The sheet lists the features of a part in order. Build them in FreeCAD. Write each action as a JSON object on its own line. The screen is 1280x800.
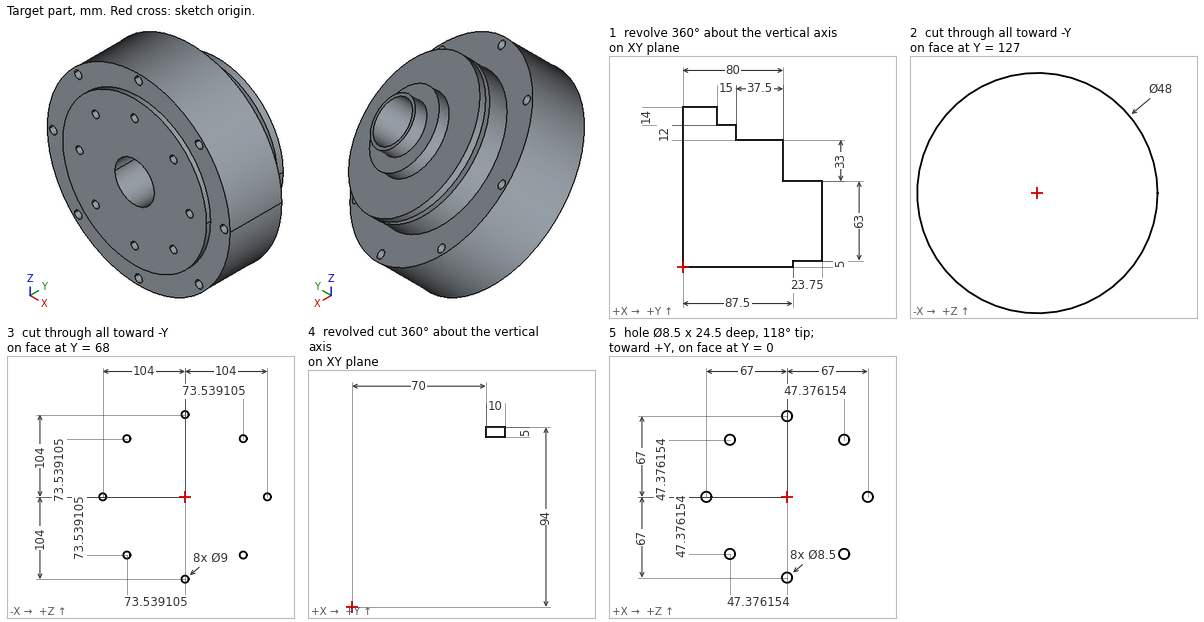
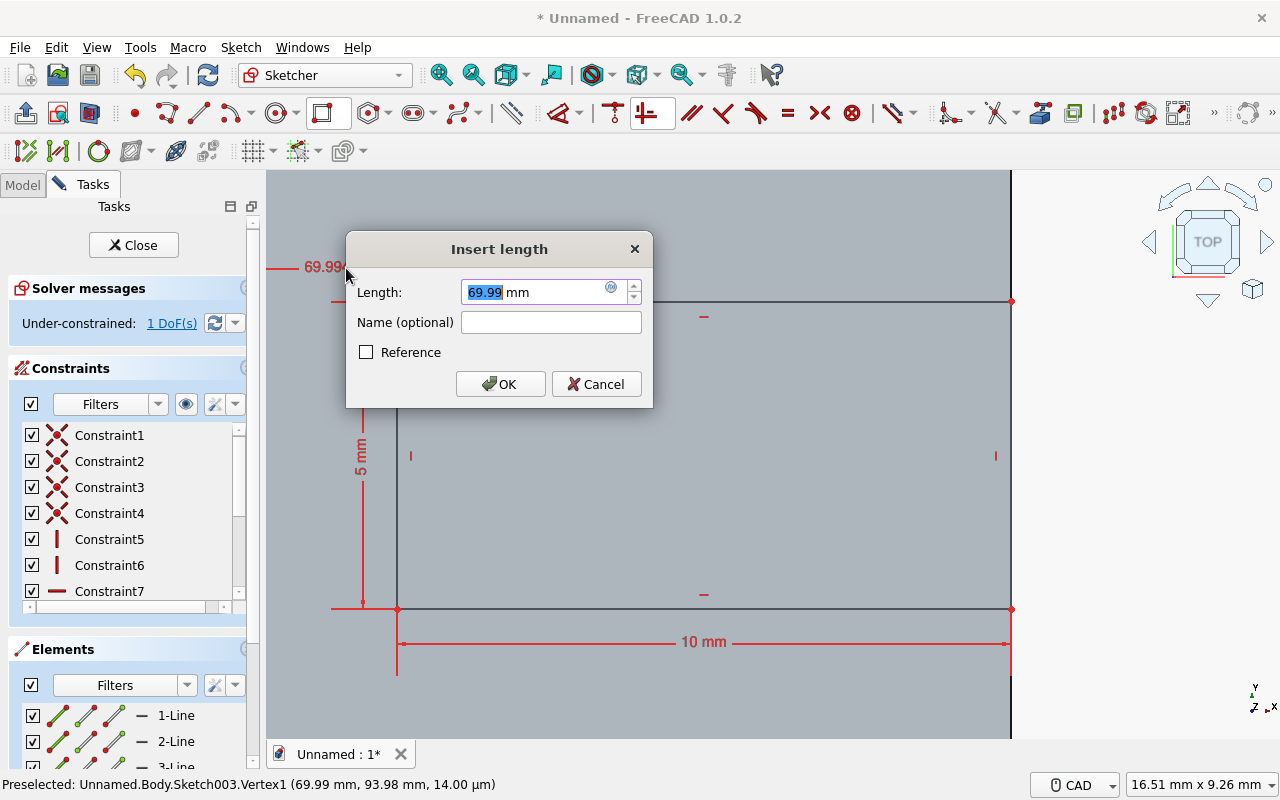
{"action": "type", "text": "70"}
{"action": "key", "text": "Return"}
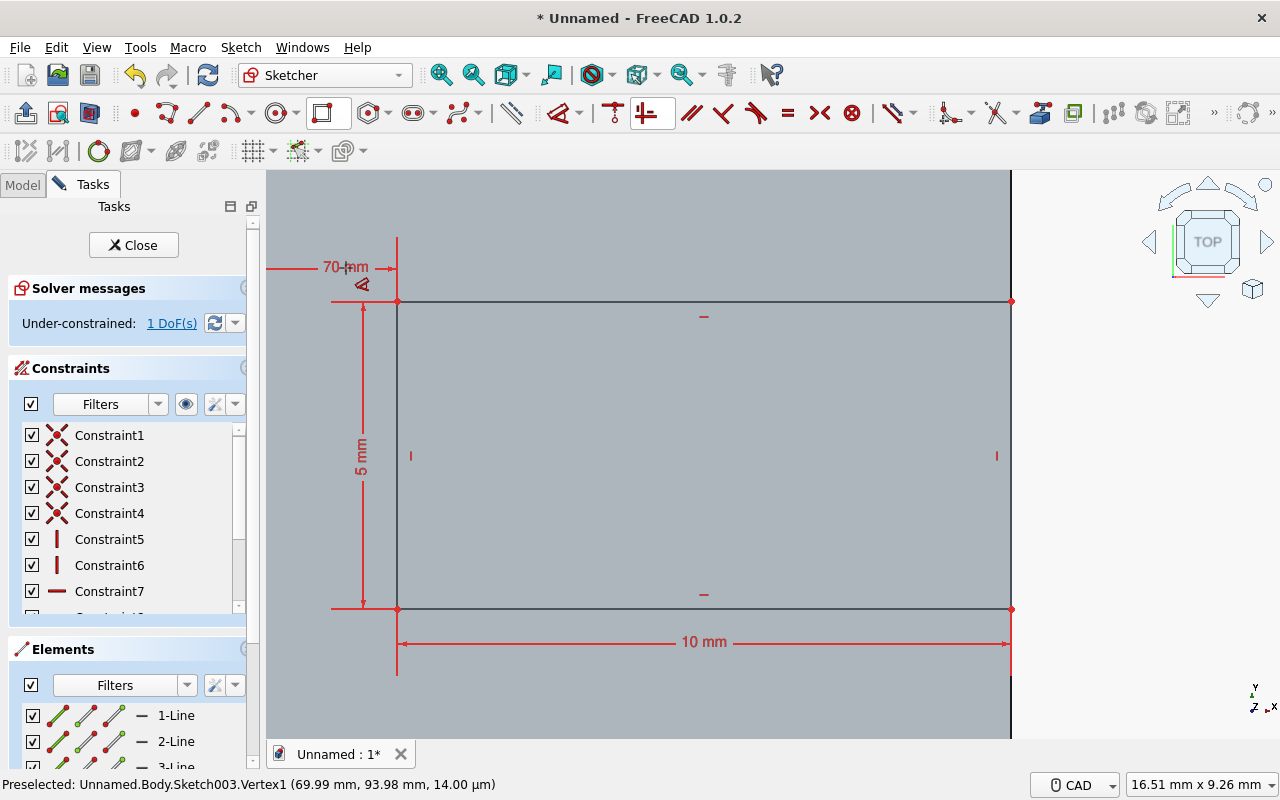
{"action": "left_click", "coordinate": [397, 302]}
{"action": "left_click", "coordinate": [431, 507]}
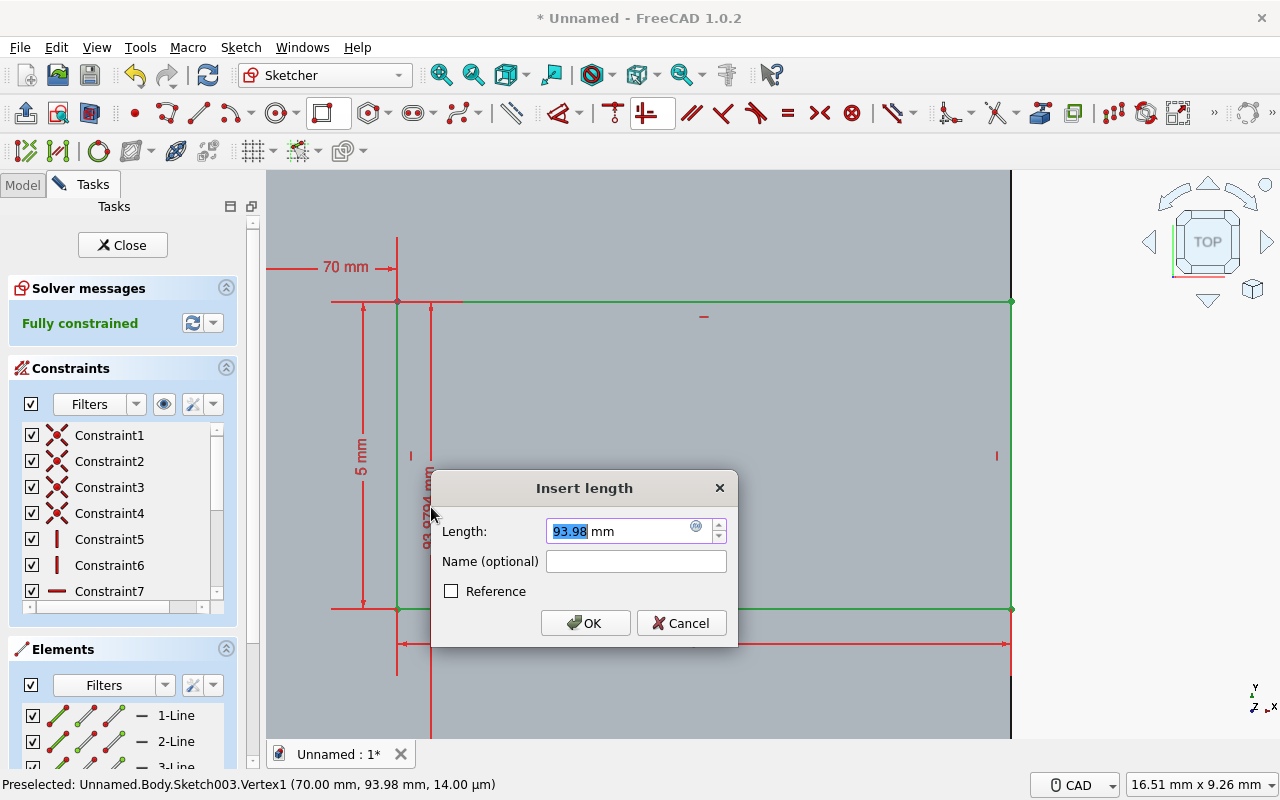
{"action": "type", "text": "94"}
{"action": "key", "text": "Return"}
{"action": "key", "text": "Escape"}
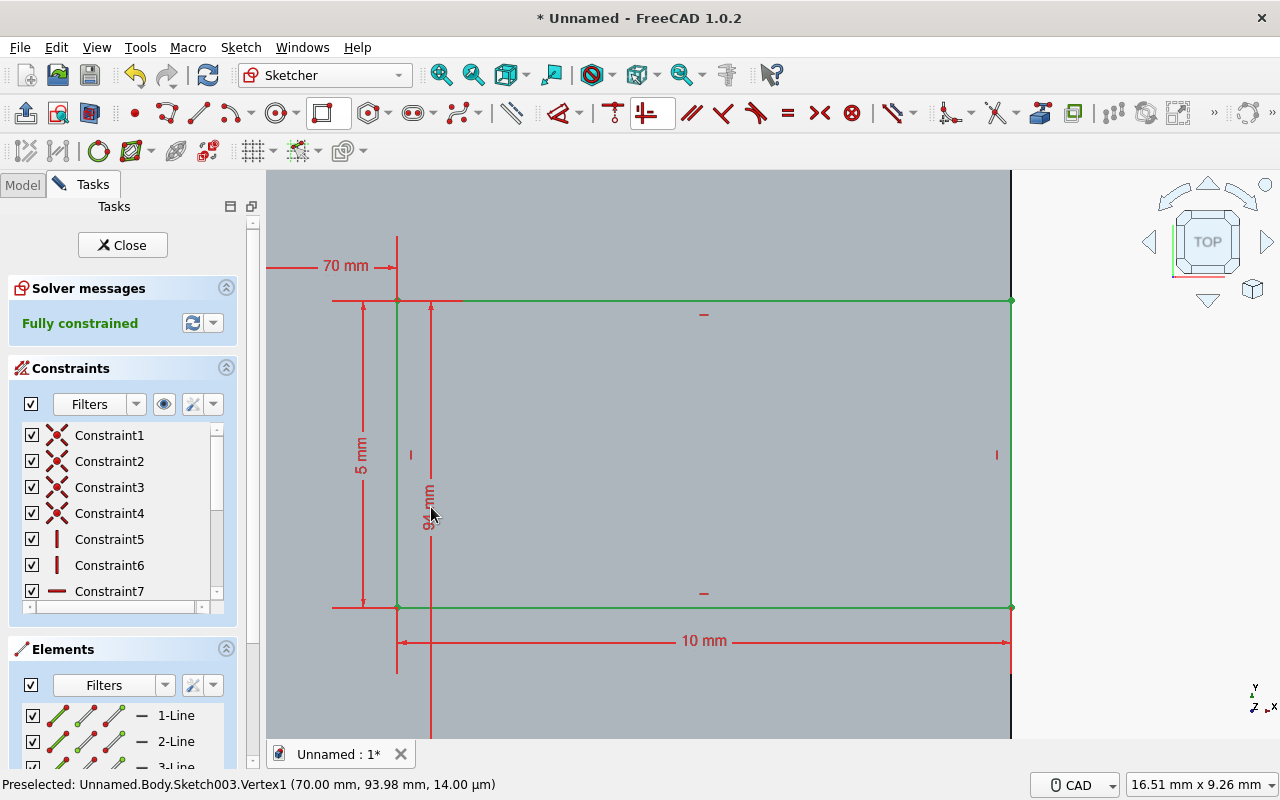
{"action": "left_click", "coordinate": [123, 245]}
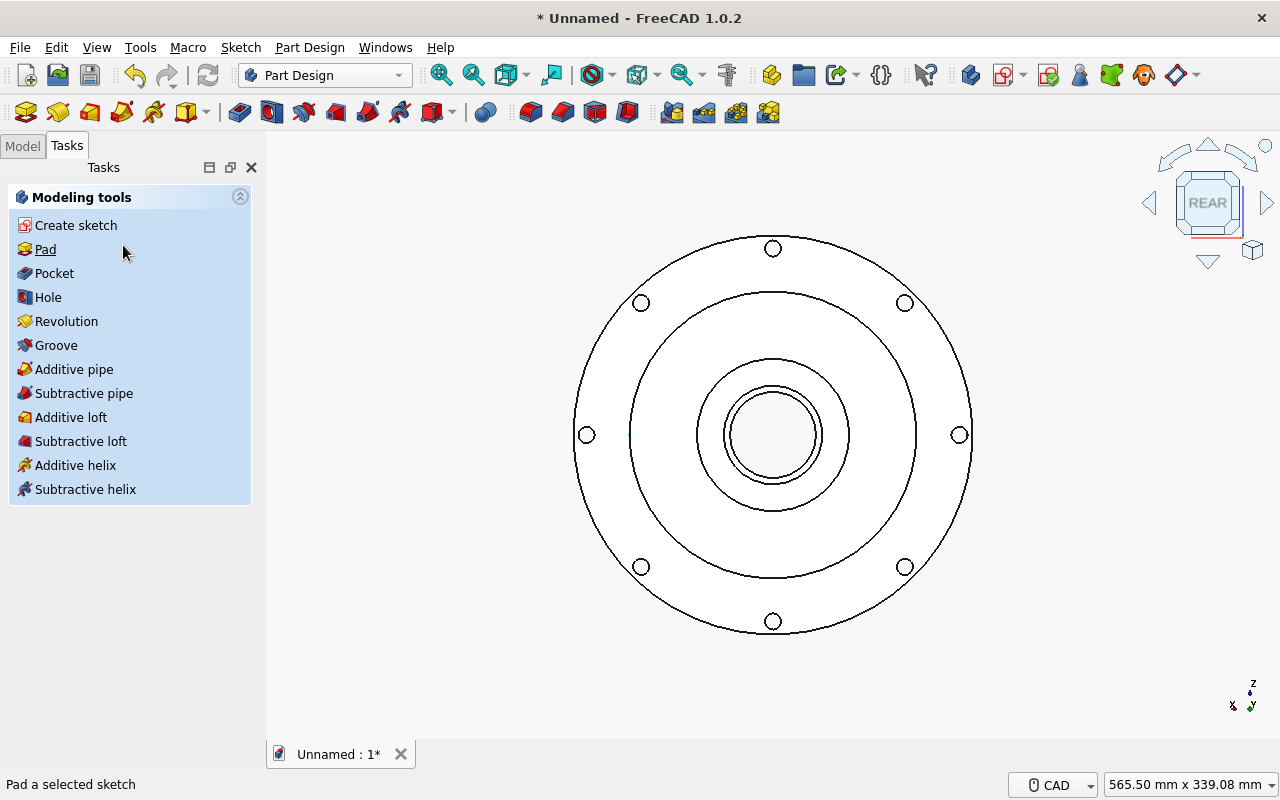
{"action": "left_click", "coordinate": [304, 112]}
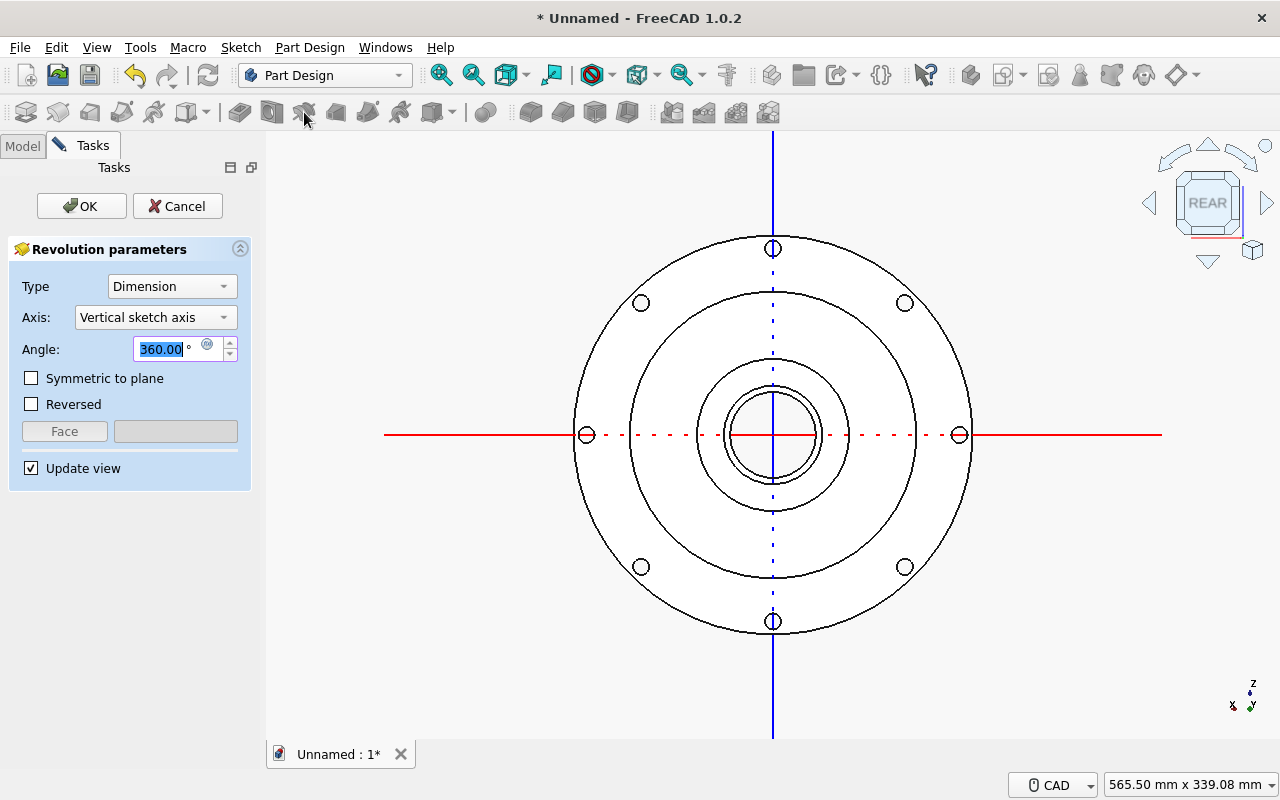
{"action": "left_click", "coordinate": [82, 206]}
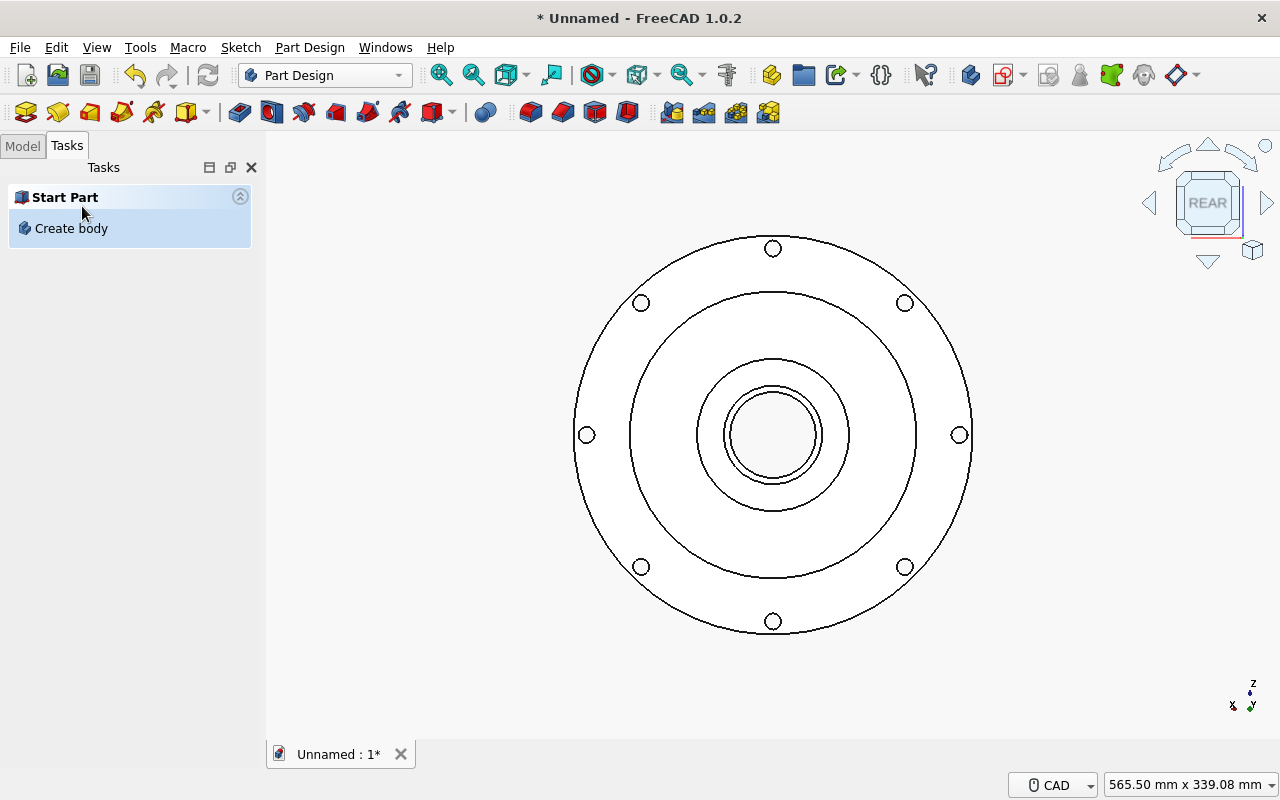
{"action": "key", "text": "0"}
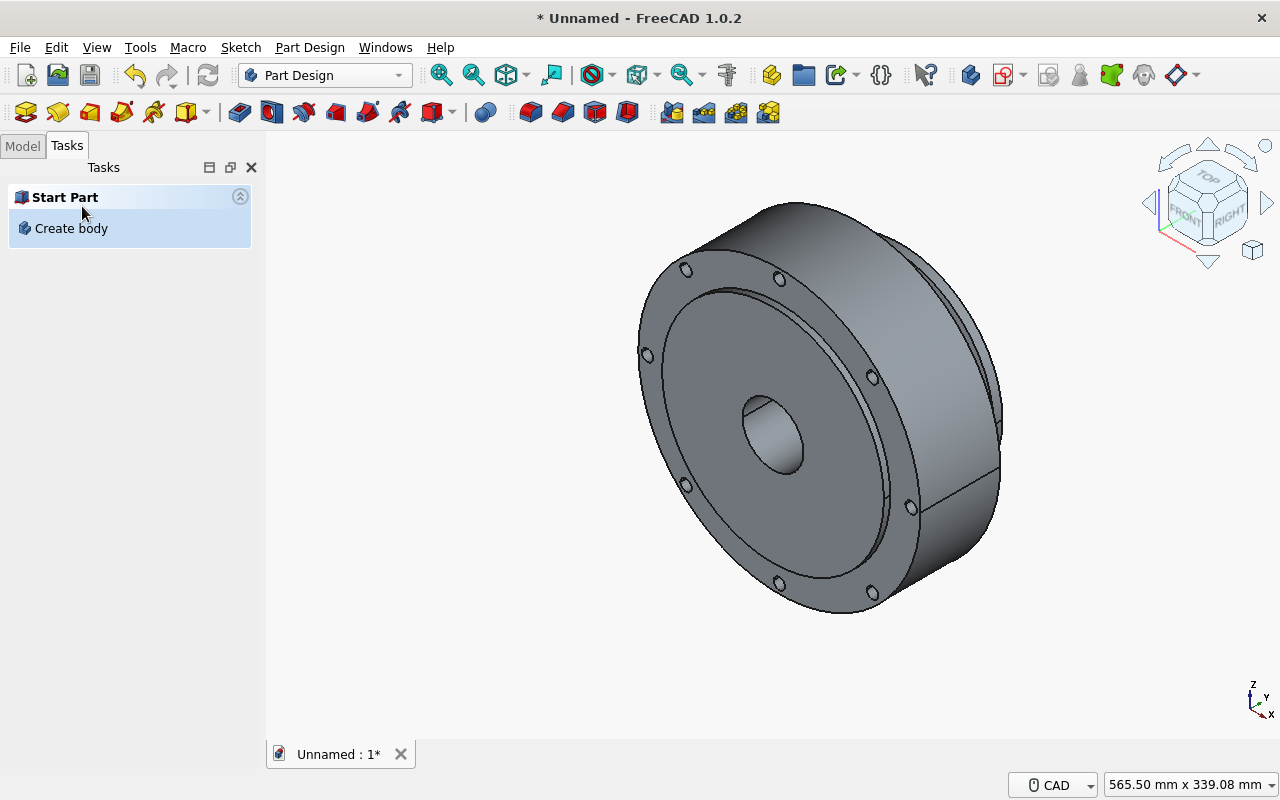
{"action": "left_click", "coordinate": [442, 76]}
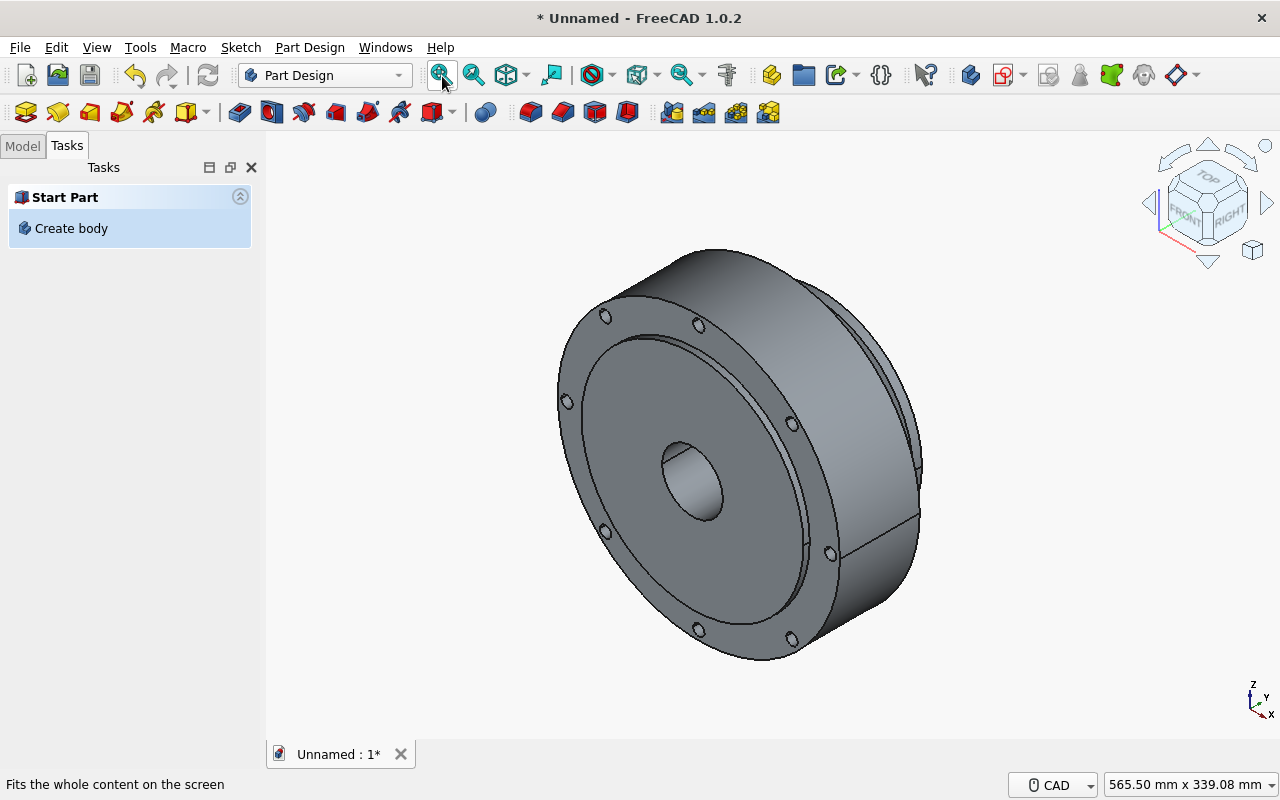
{"action": "left_click", "coordinate": [756, 554]}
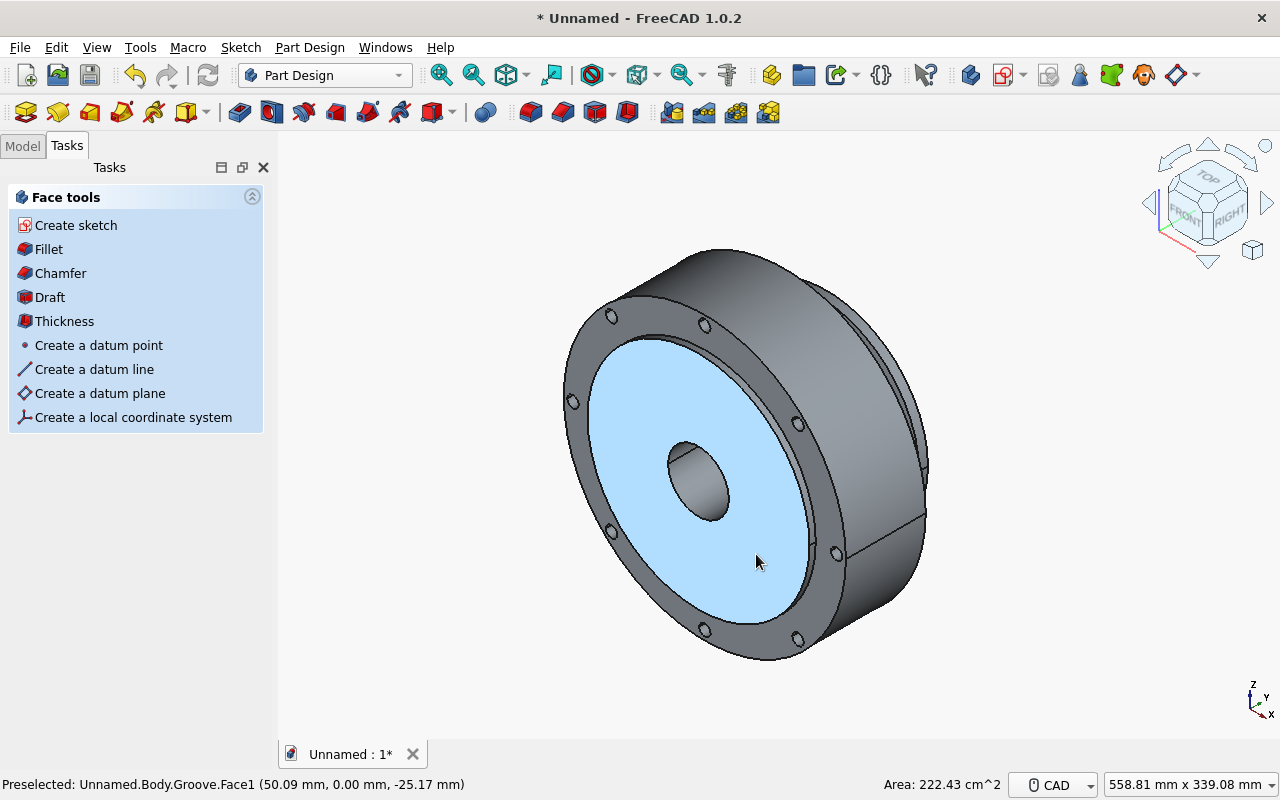
{"action": "left_click", "coordinate": [1004, 76]}